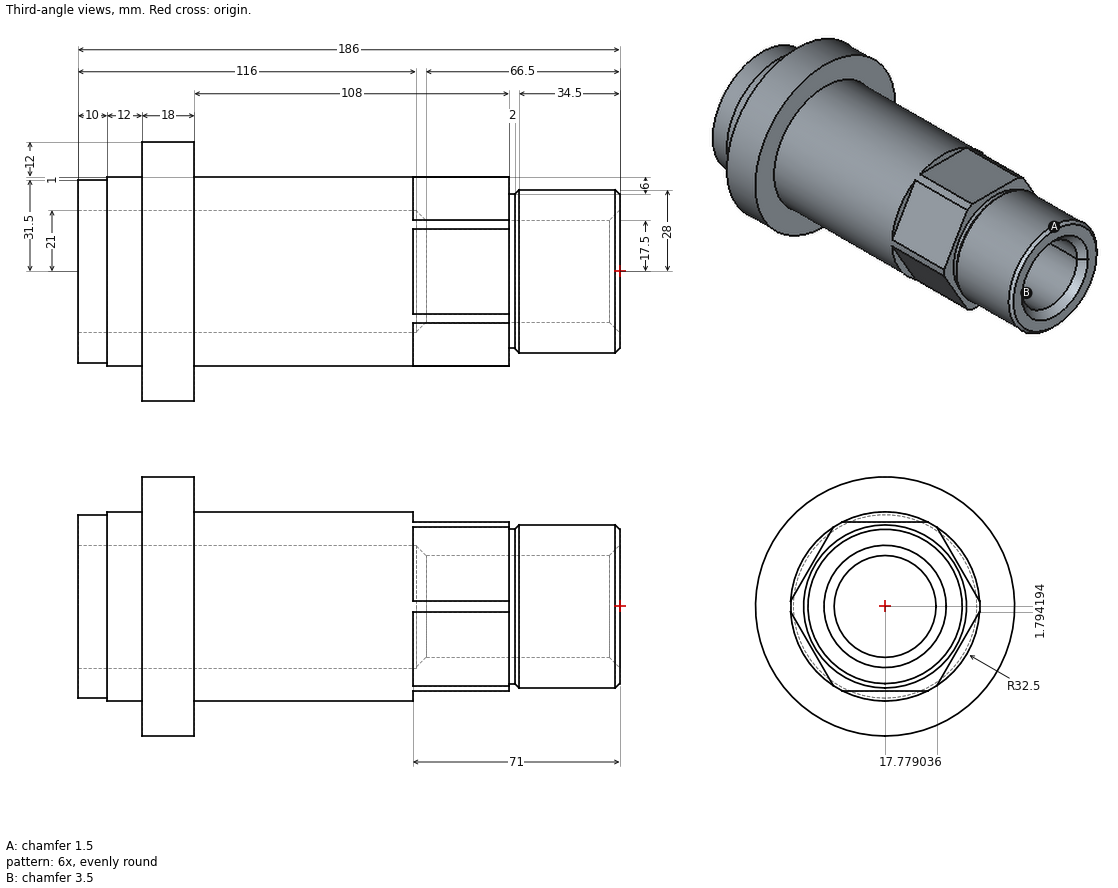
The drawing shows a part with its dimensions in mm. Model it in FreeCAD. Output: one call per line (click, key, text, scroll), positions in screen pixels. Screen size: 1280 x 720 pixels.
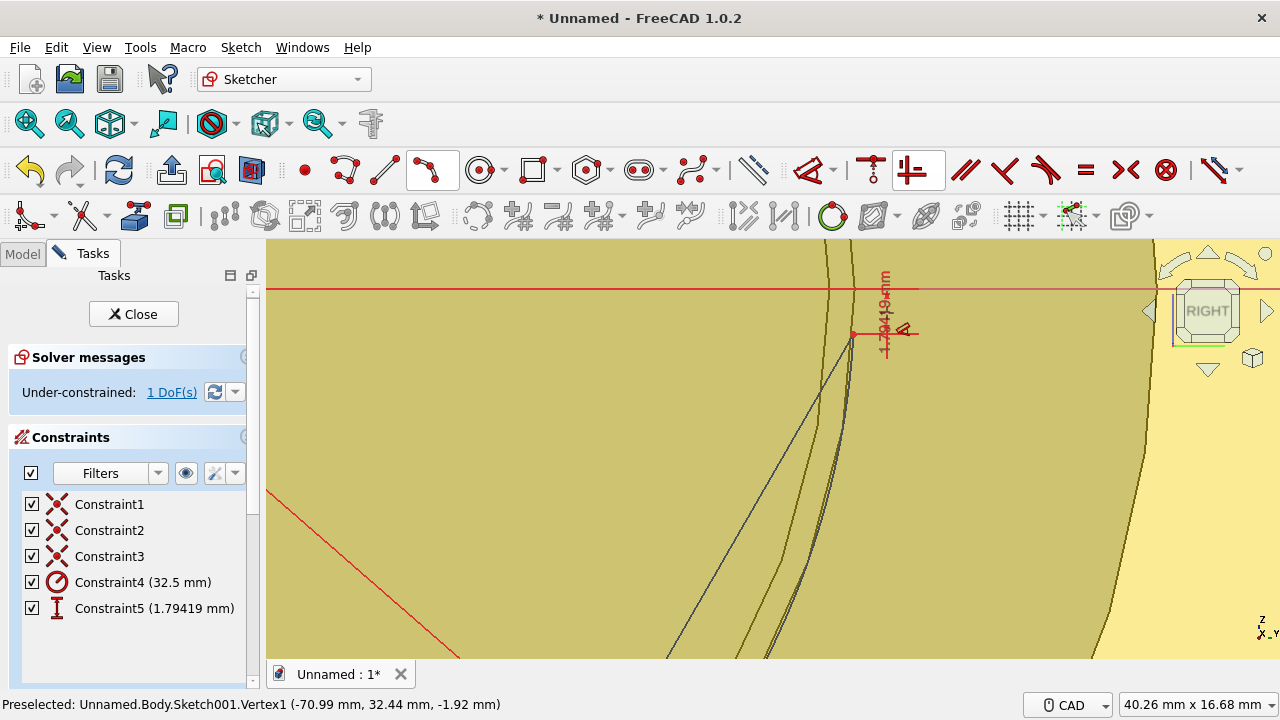
scroll(856, 343, down, 5)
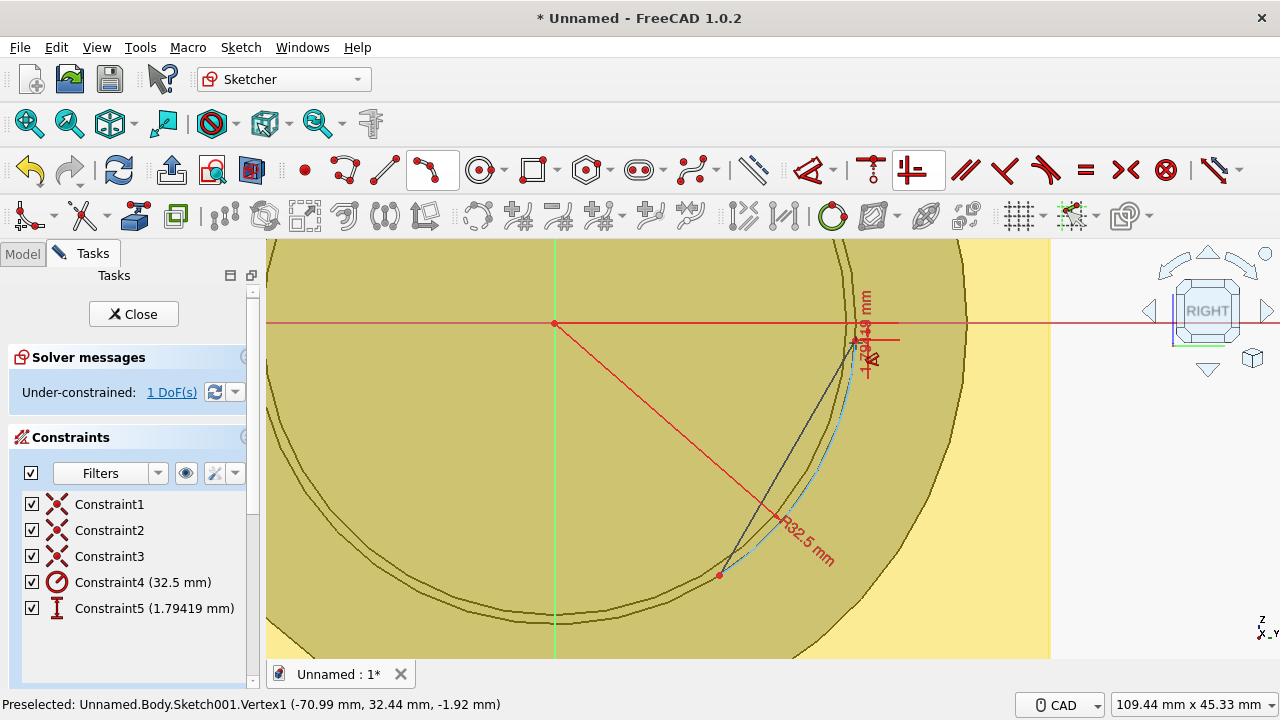
click(720, 575)
click(637, 289)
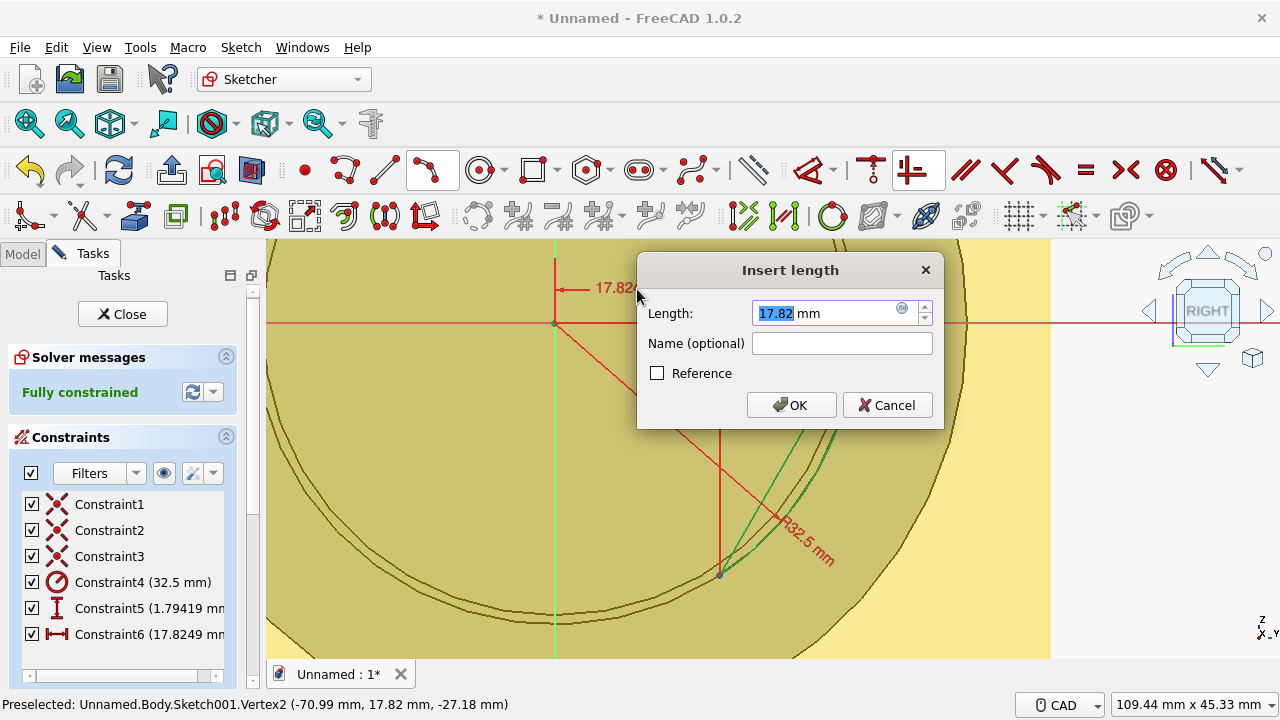
text(17.779036)
key(Return)
key(Escape)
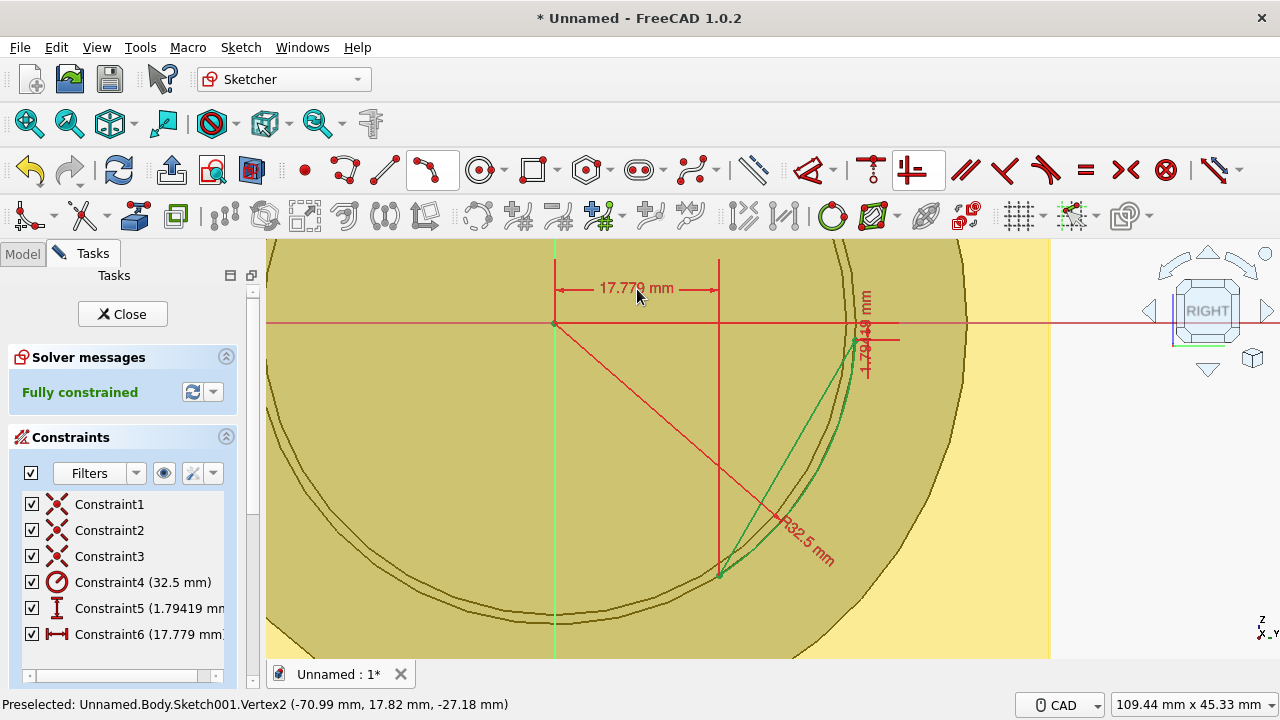
click(123, 314)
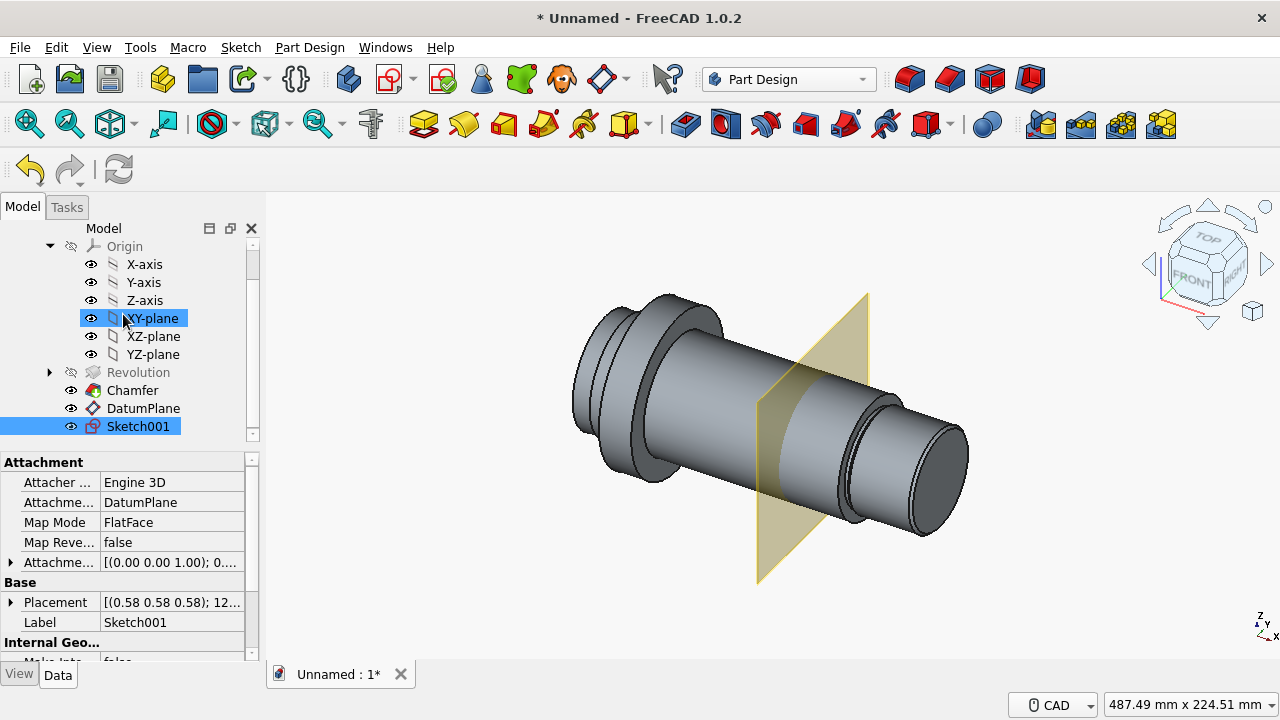
click(686, 124)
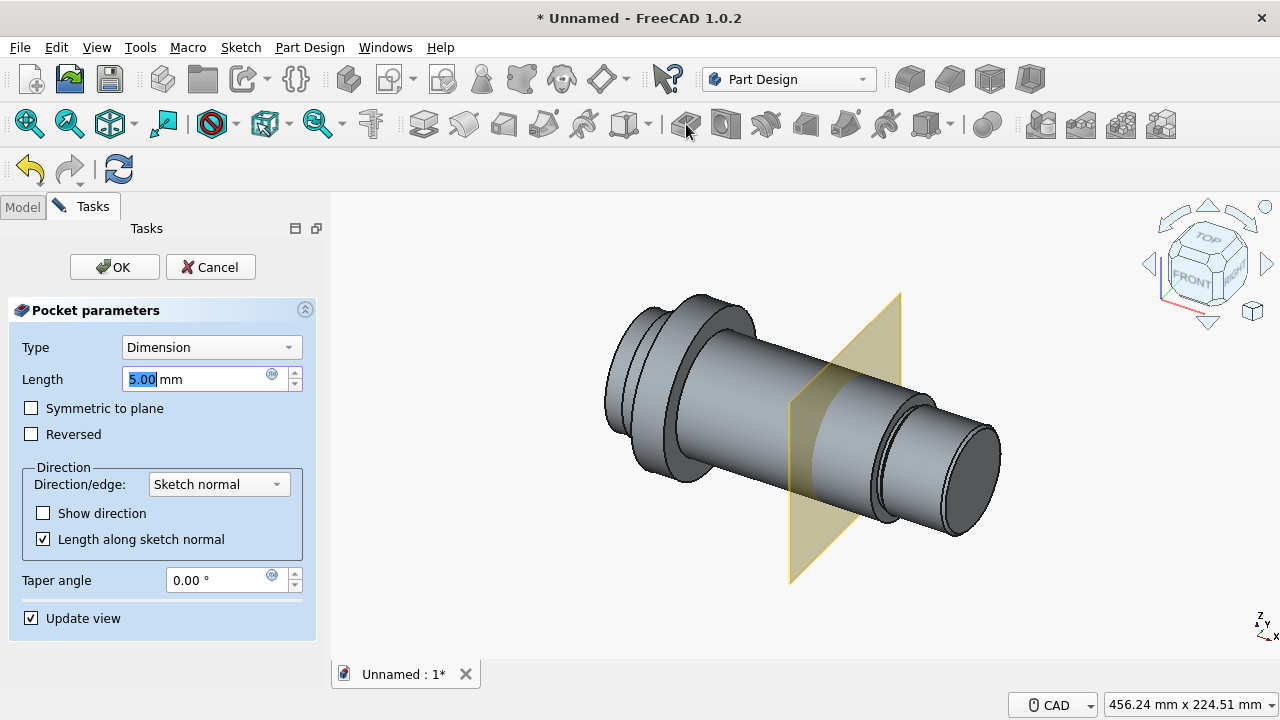
text(71)
key(Tab)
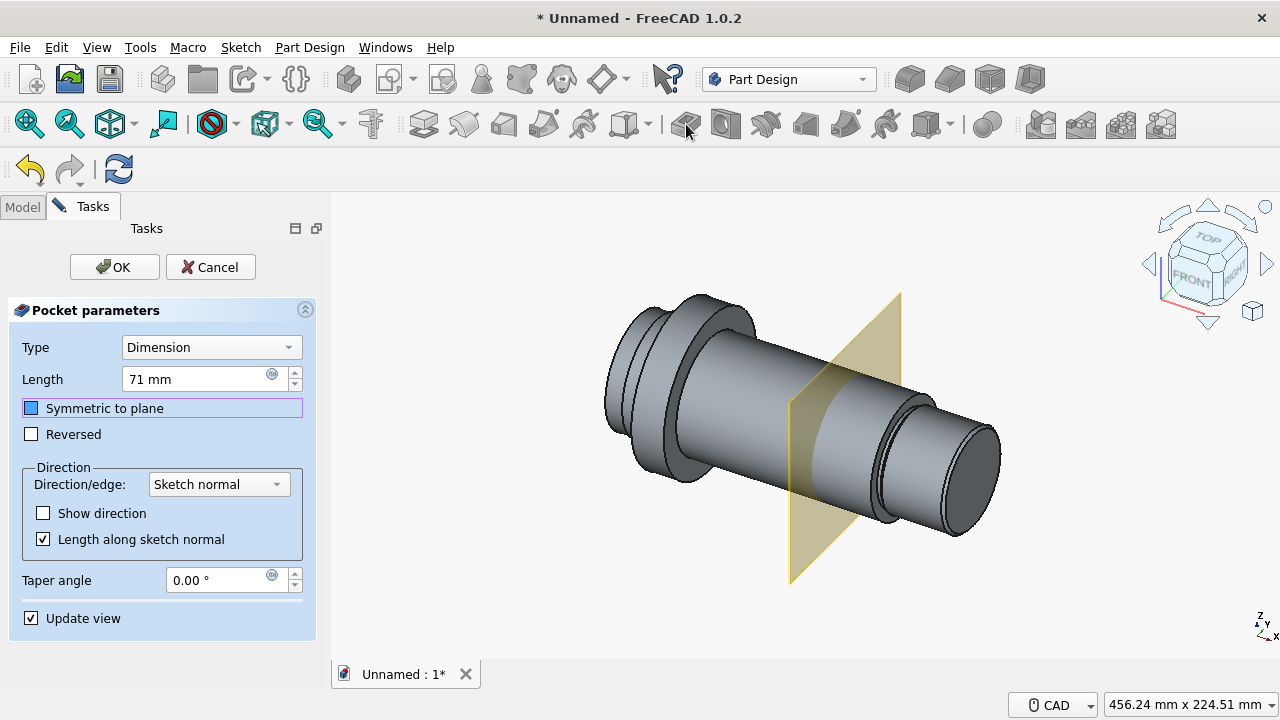
click(30, 434)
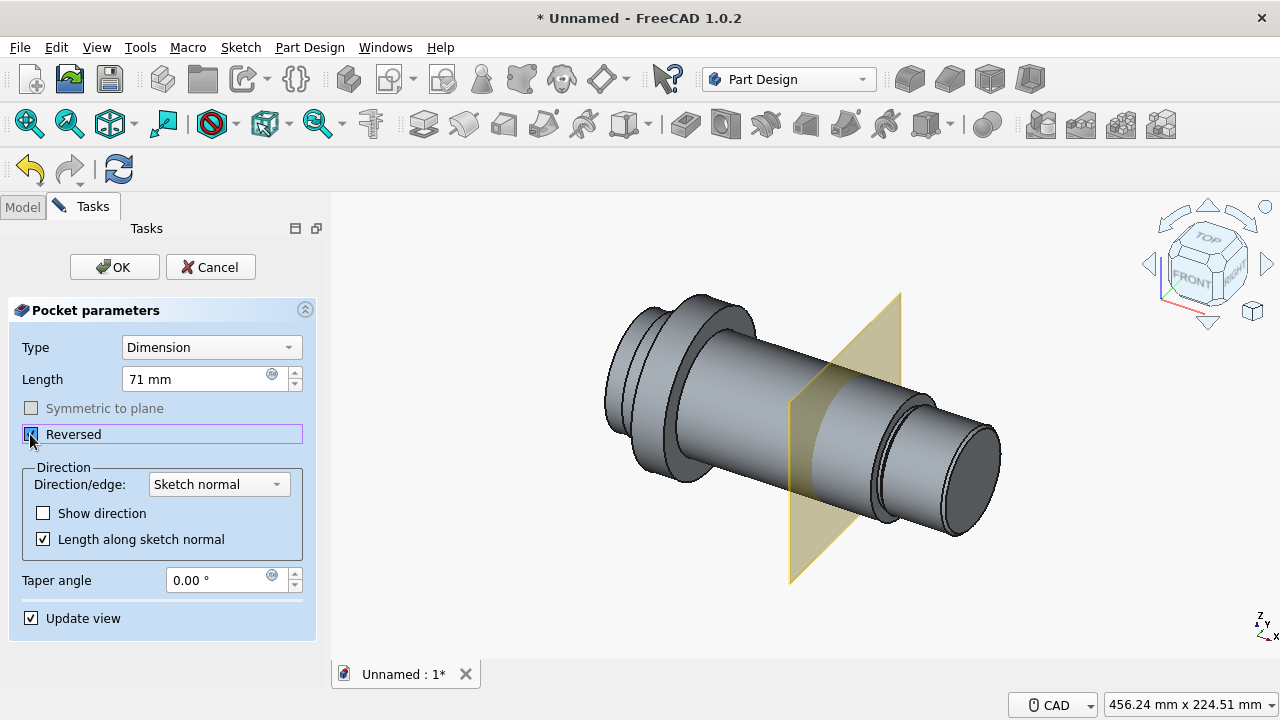
click(115, 267)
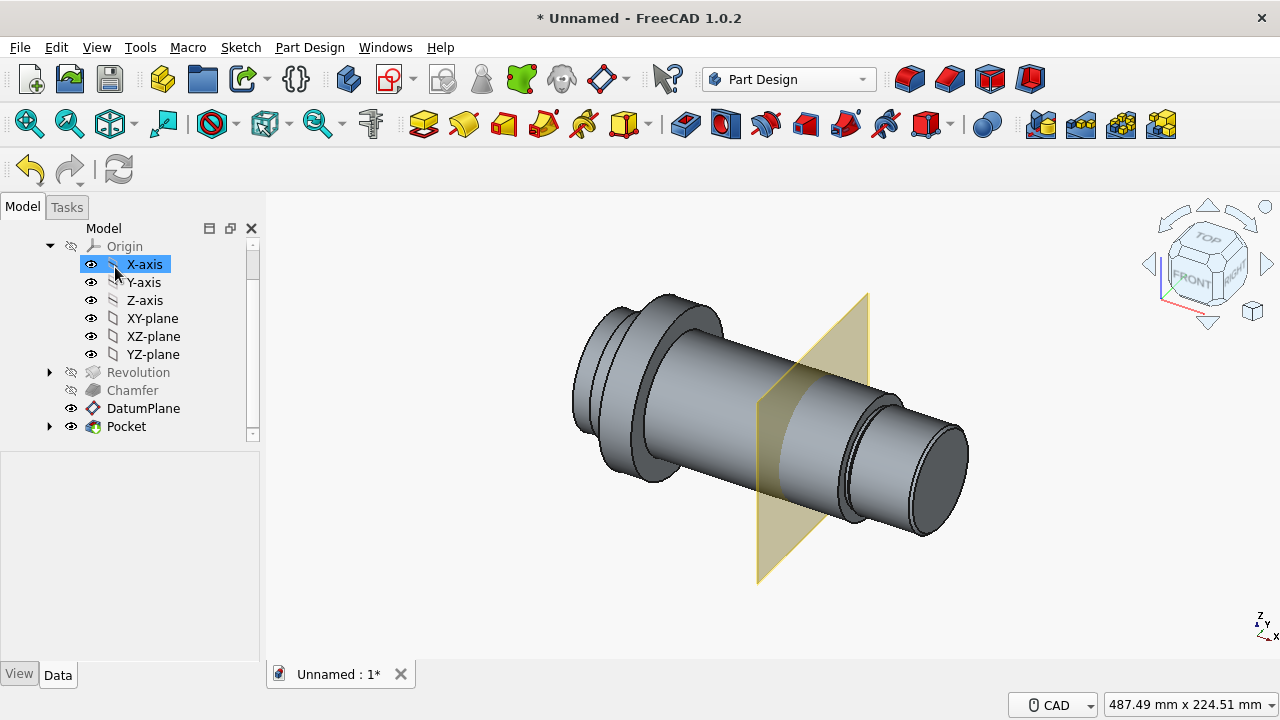
click(116, 408)
key(space)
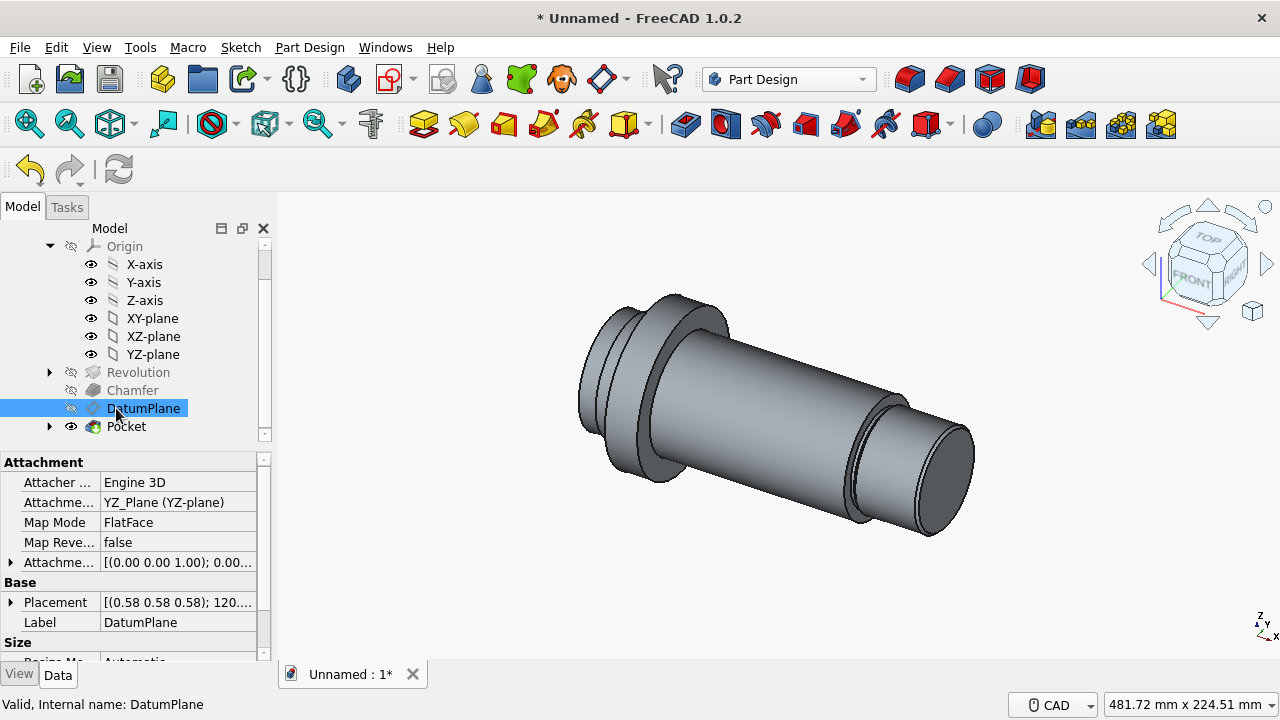
click(116, 426)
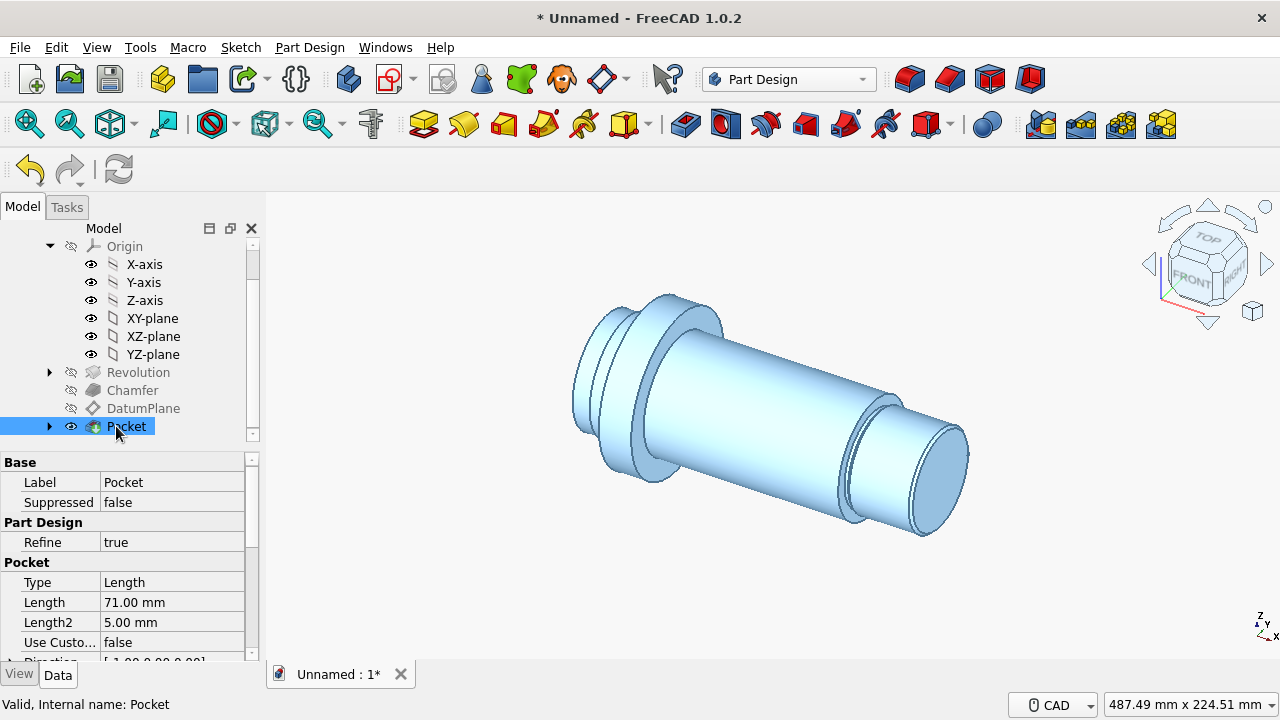
click(1122, 124)